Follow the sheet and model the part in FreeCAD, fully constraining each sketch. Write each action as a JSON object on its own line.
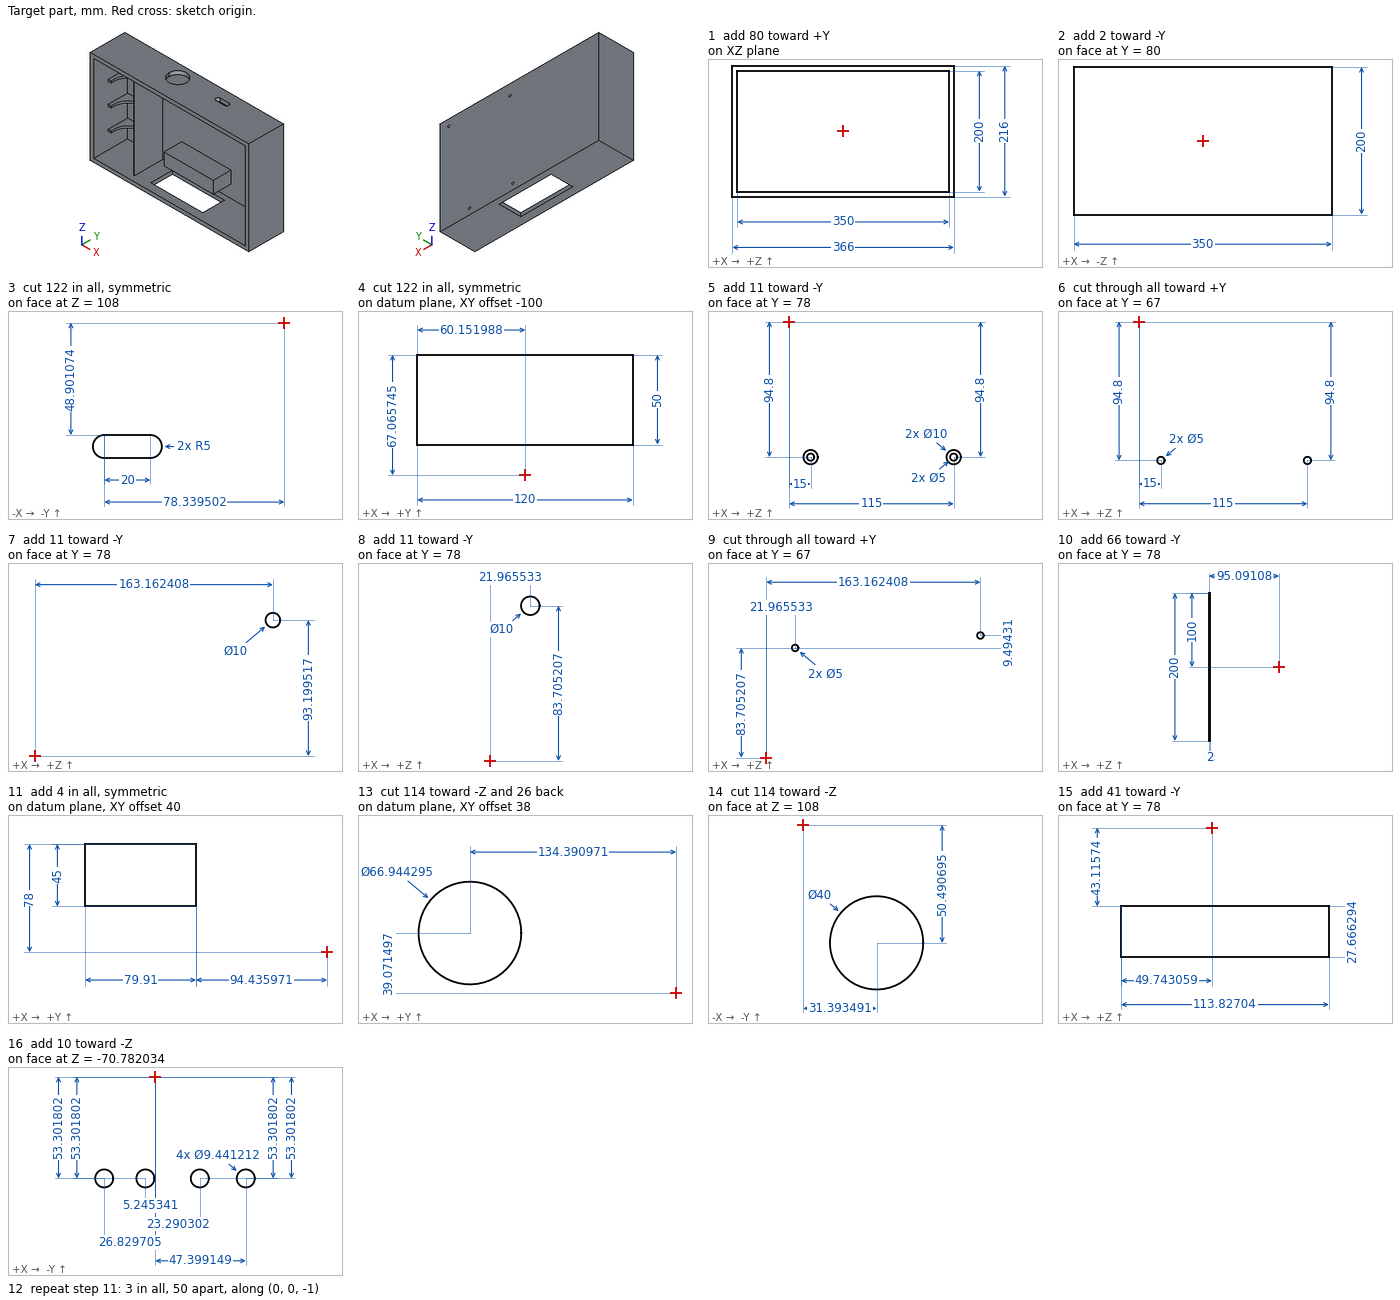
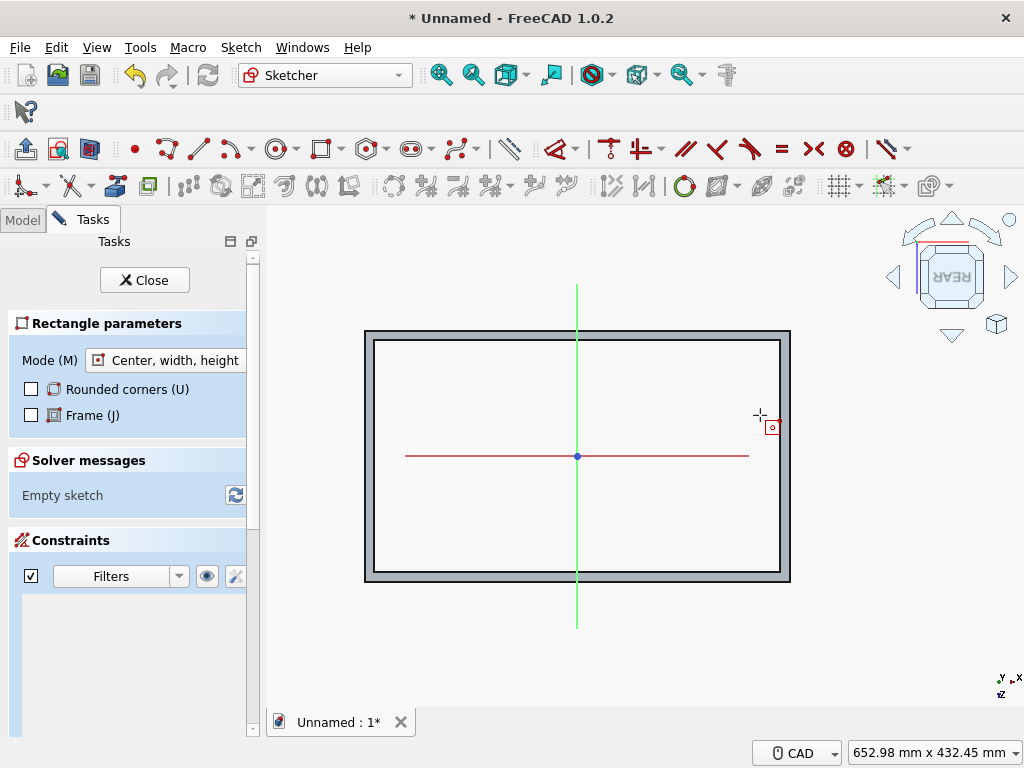
{"action": "left_click", "coordinate": [577, 456]}
{"action": "mouse_move", "coordinate": [780, 340]}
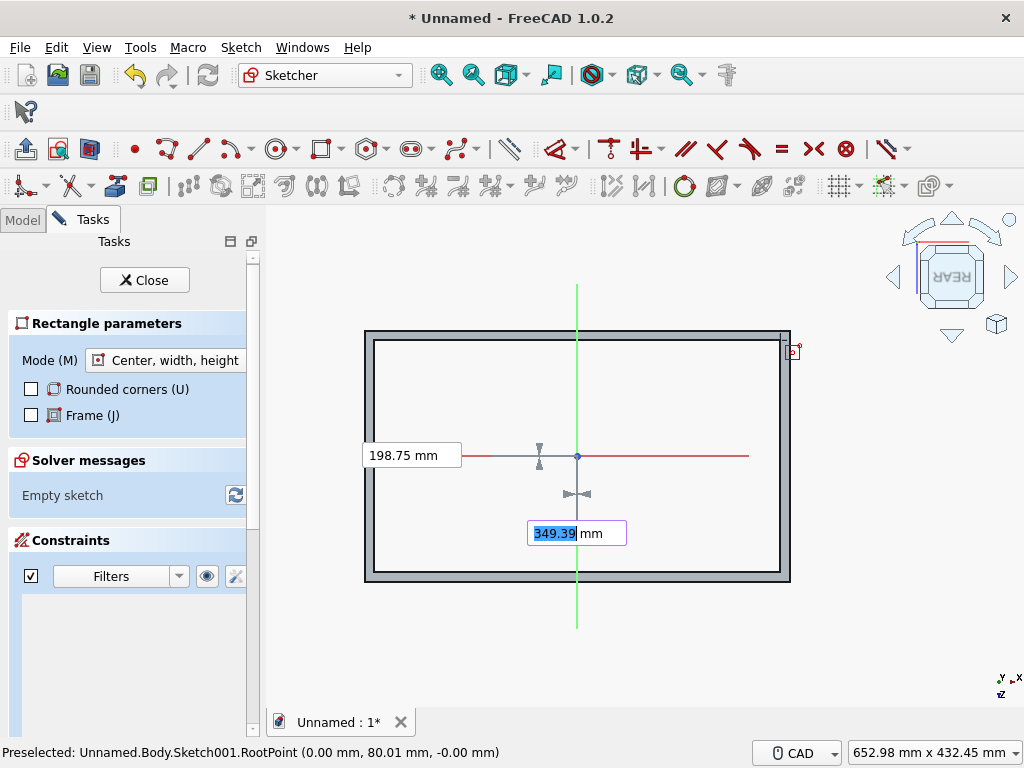
{"action": "type", "text": "350"}
{"action": "key", "text": "Tab"}
{"action": "type", "text": "200"}
{"action": "key", "text": "Return"}
{"action": "key", "text": "Escape"}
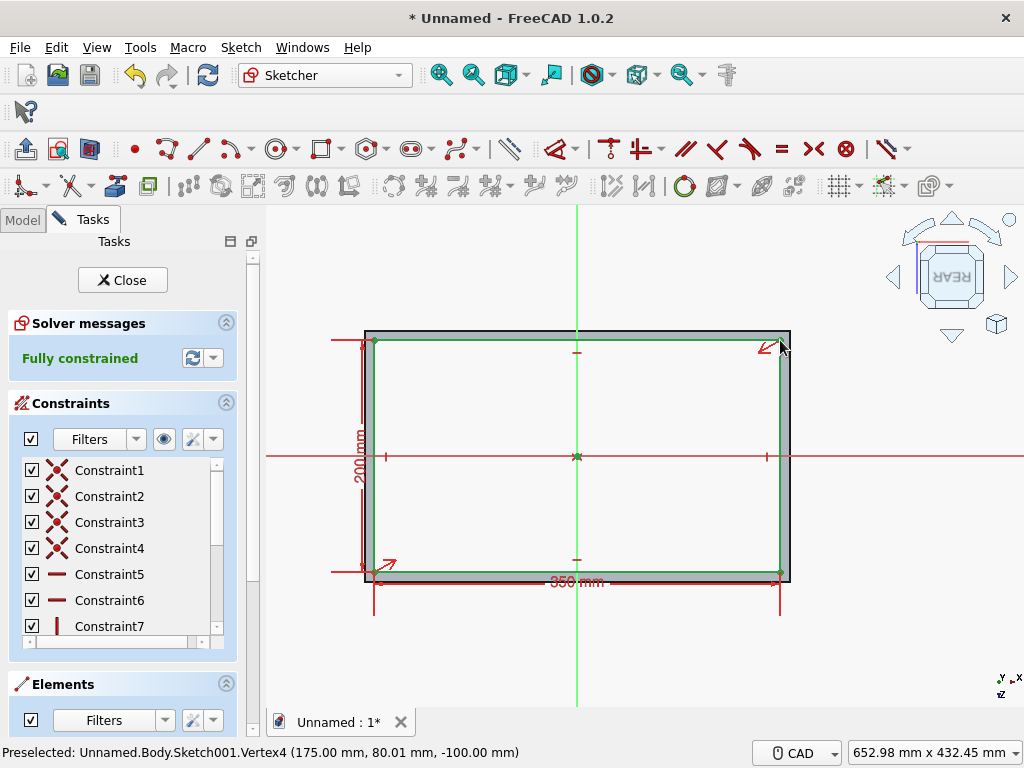
{"action": "left_click", "coordinate": [123, 280]}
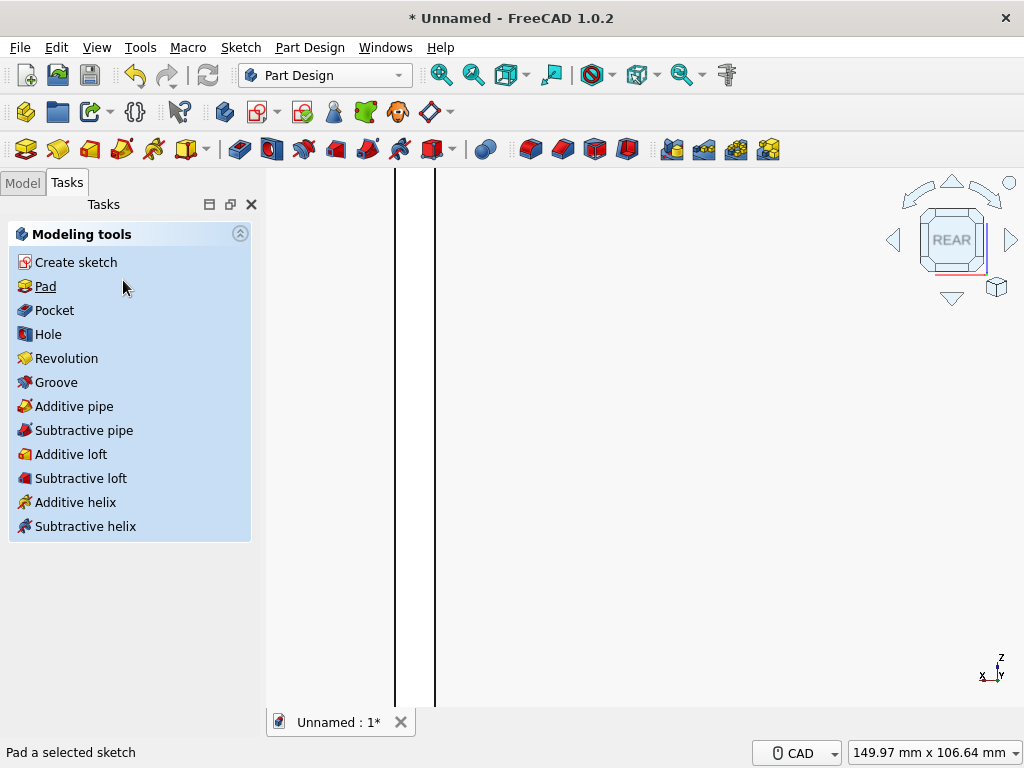
{"action": "left_click", "coordinate": [26, 150]}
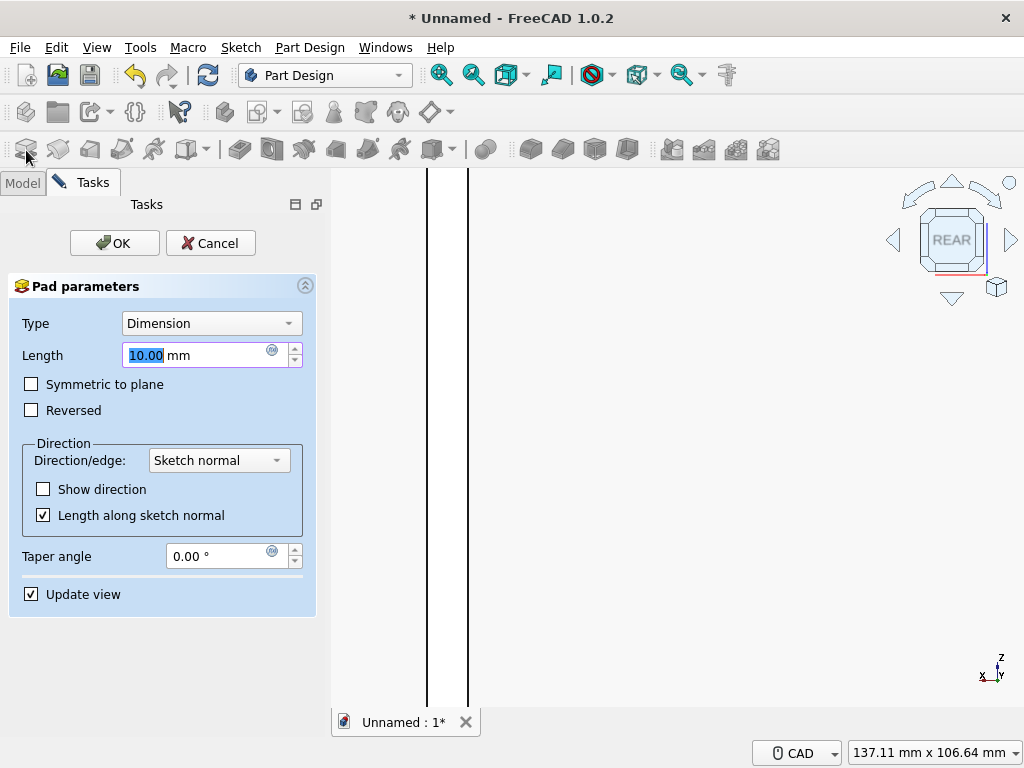
{"action": "type", "text": "2"}
{"action": "key", "text": "Tab"}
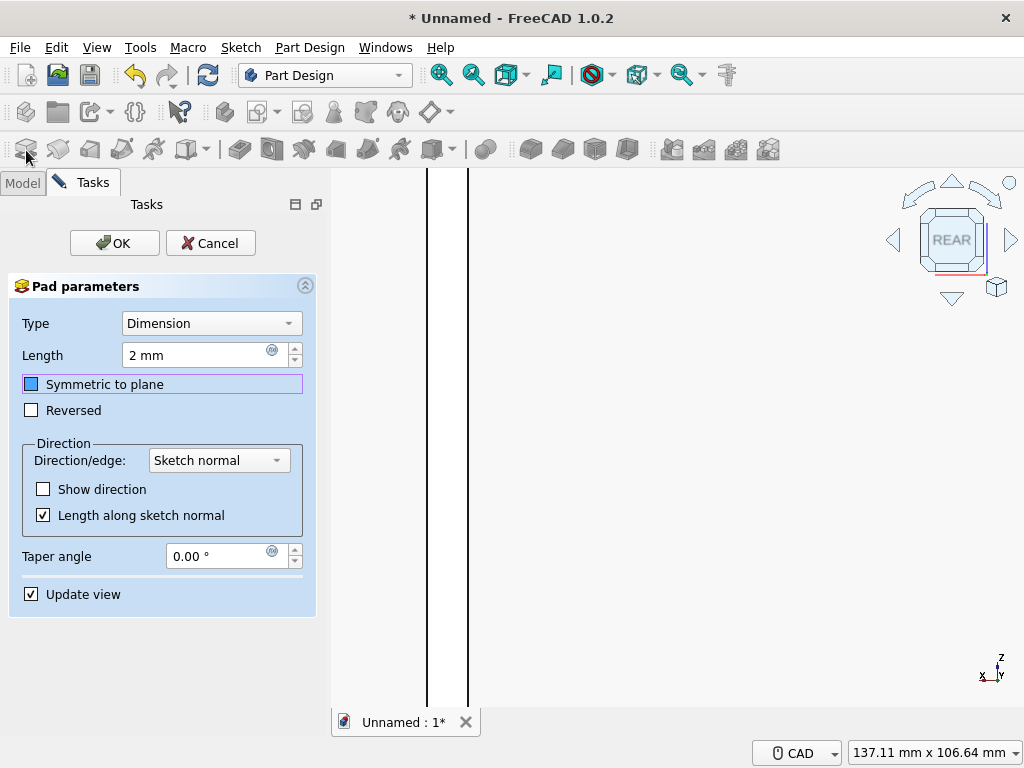
{"action": "left_click", "coordinate": [30, 410]}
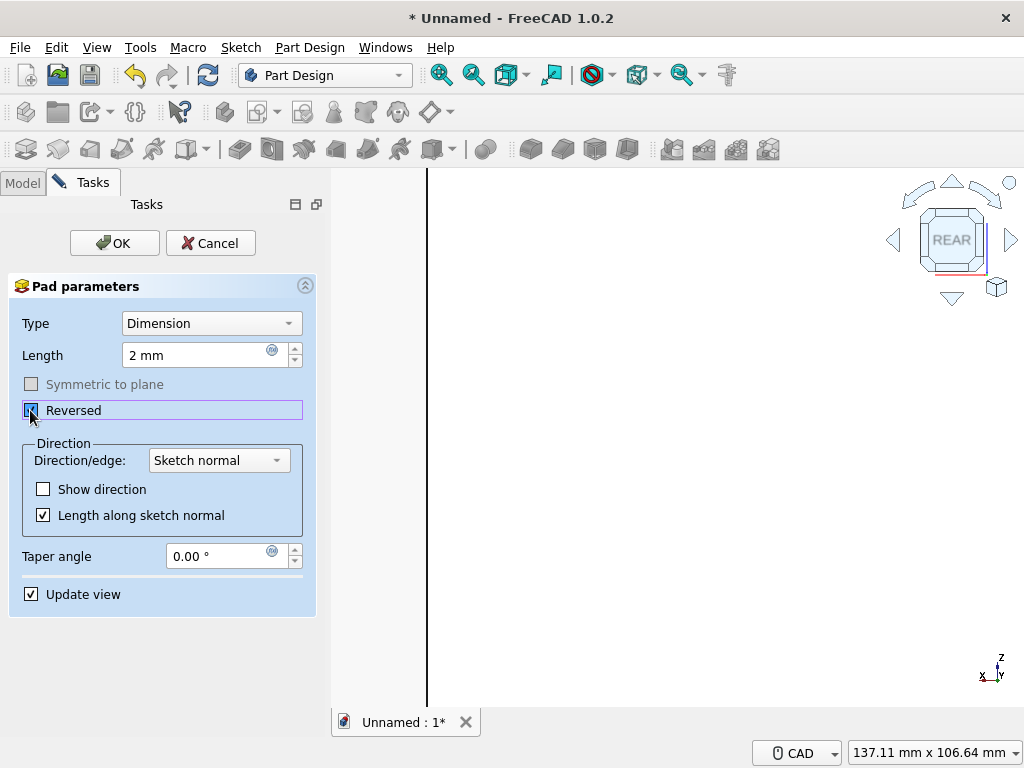
{"action": "left_click", "coordinate": [115, 243]}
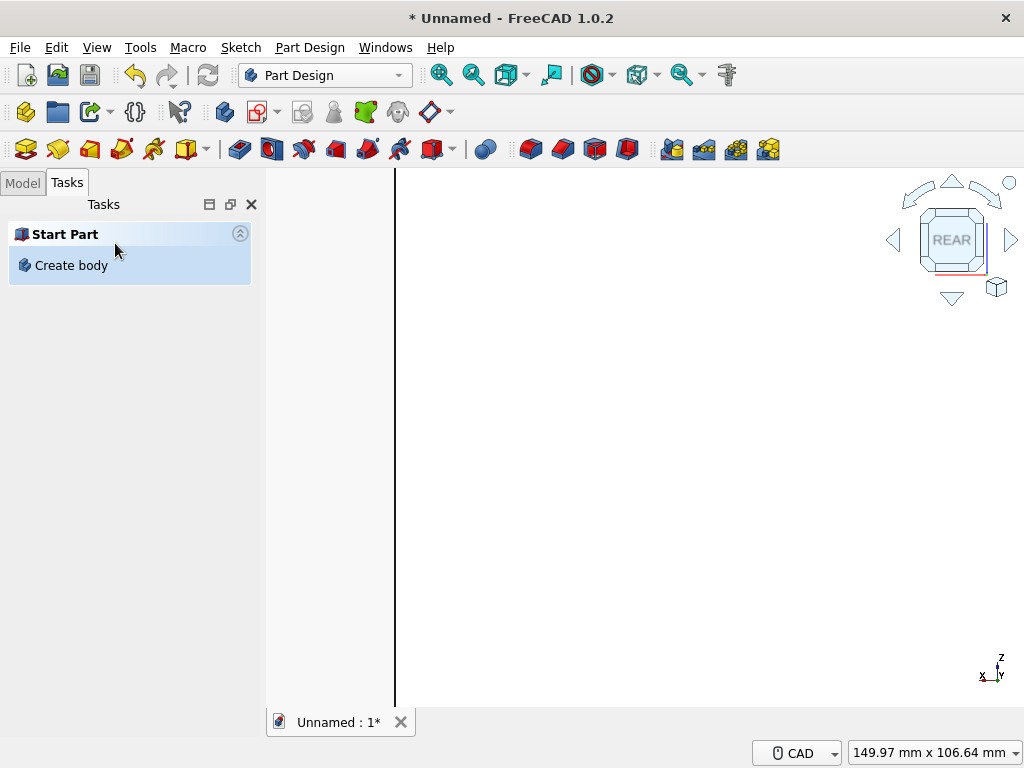
{"action": "key", "text": "v f"}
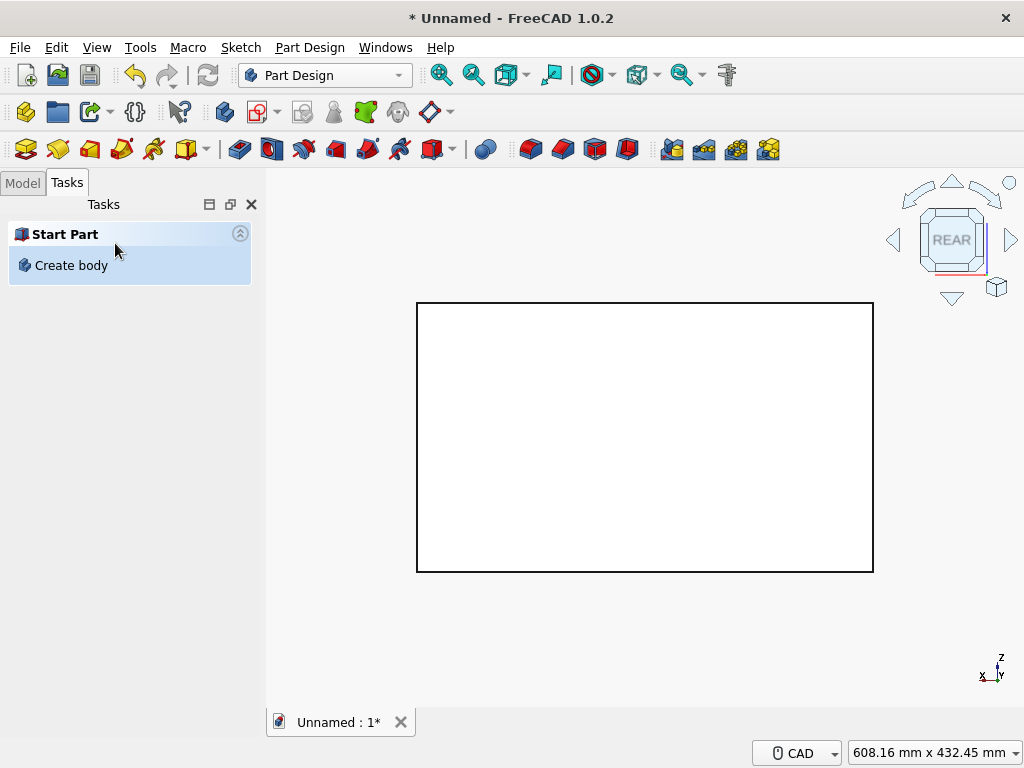
{"action": "key", "text": "0"}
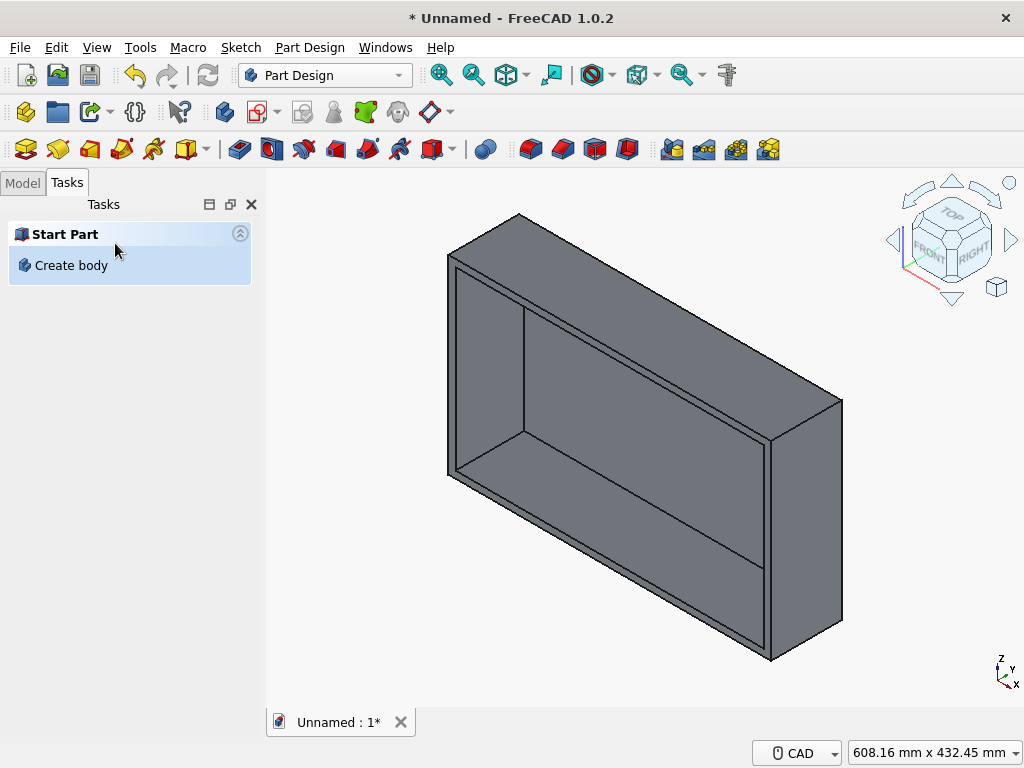
{"action": "left_click", "coordinate": [737, 380]}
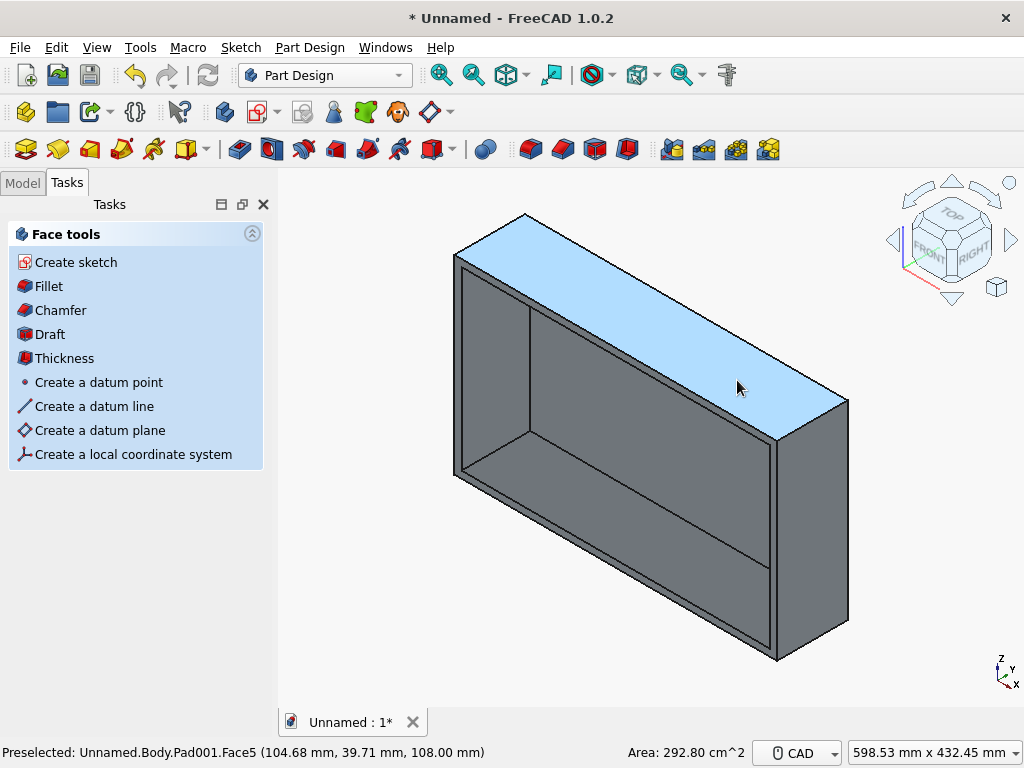
{"action": "left_click", "coordinate": [258, 112]}